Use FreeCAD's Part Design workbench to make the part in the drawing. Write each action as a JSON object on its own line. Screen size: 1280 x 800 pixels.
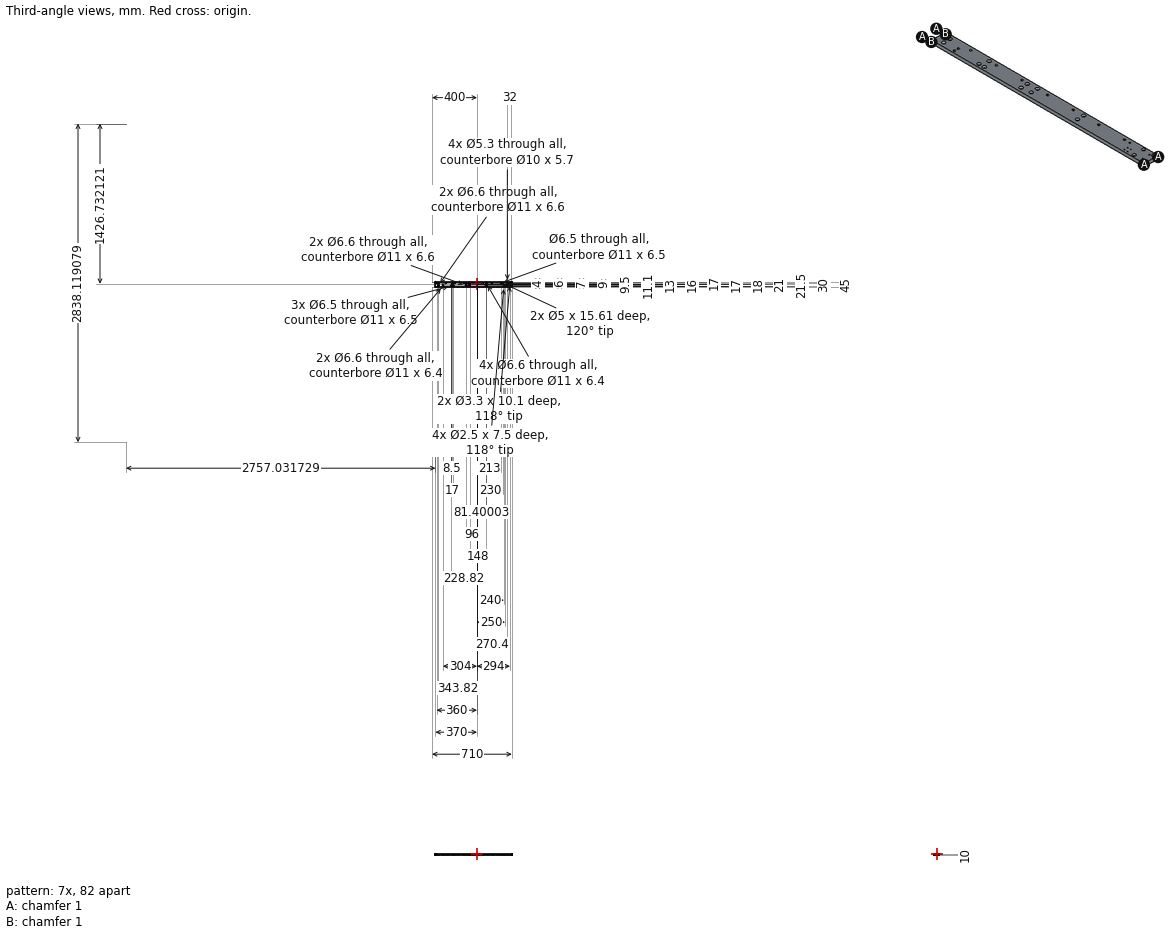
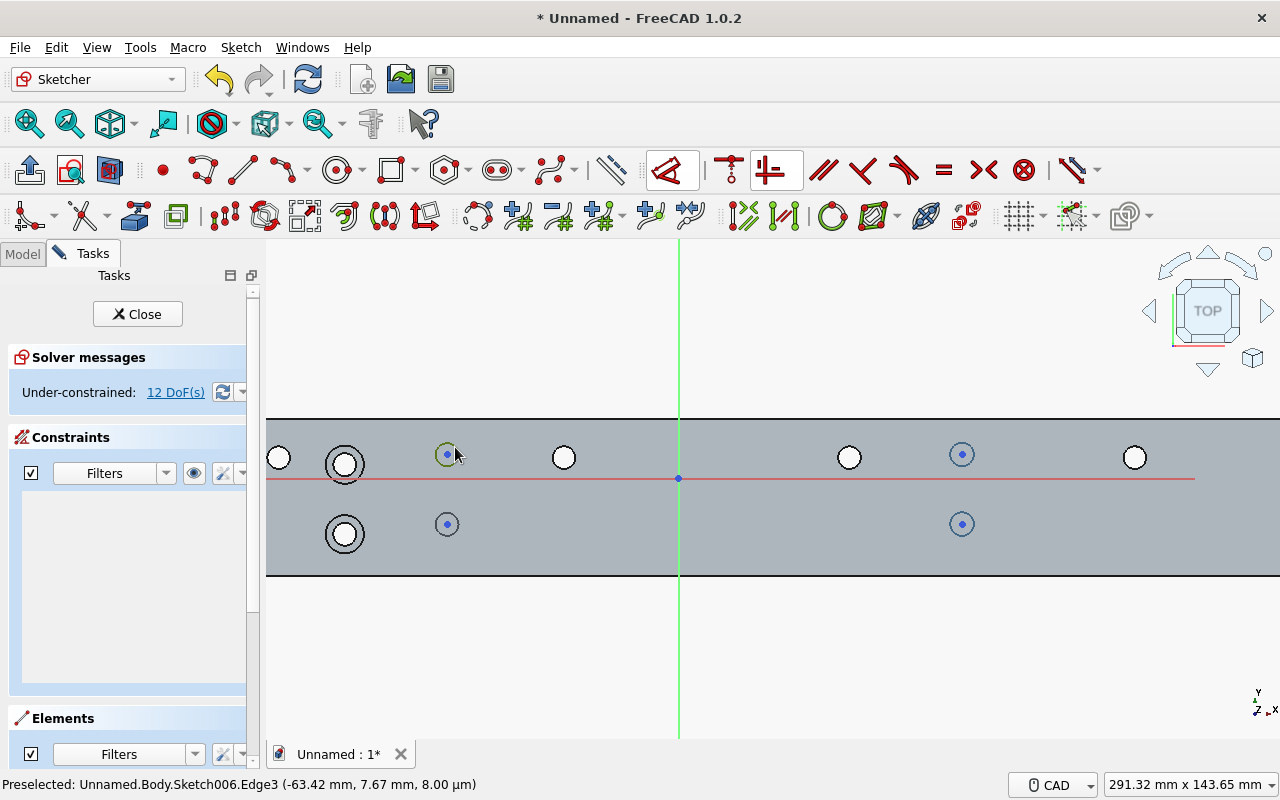
{"action": "left_click", "coordinate": [455, 516]}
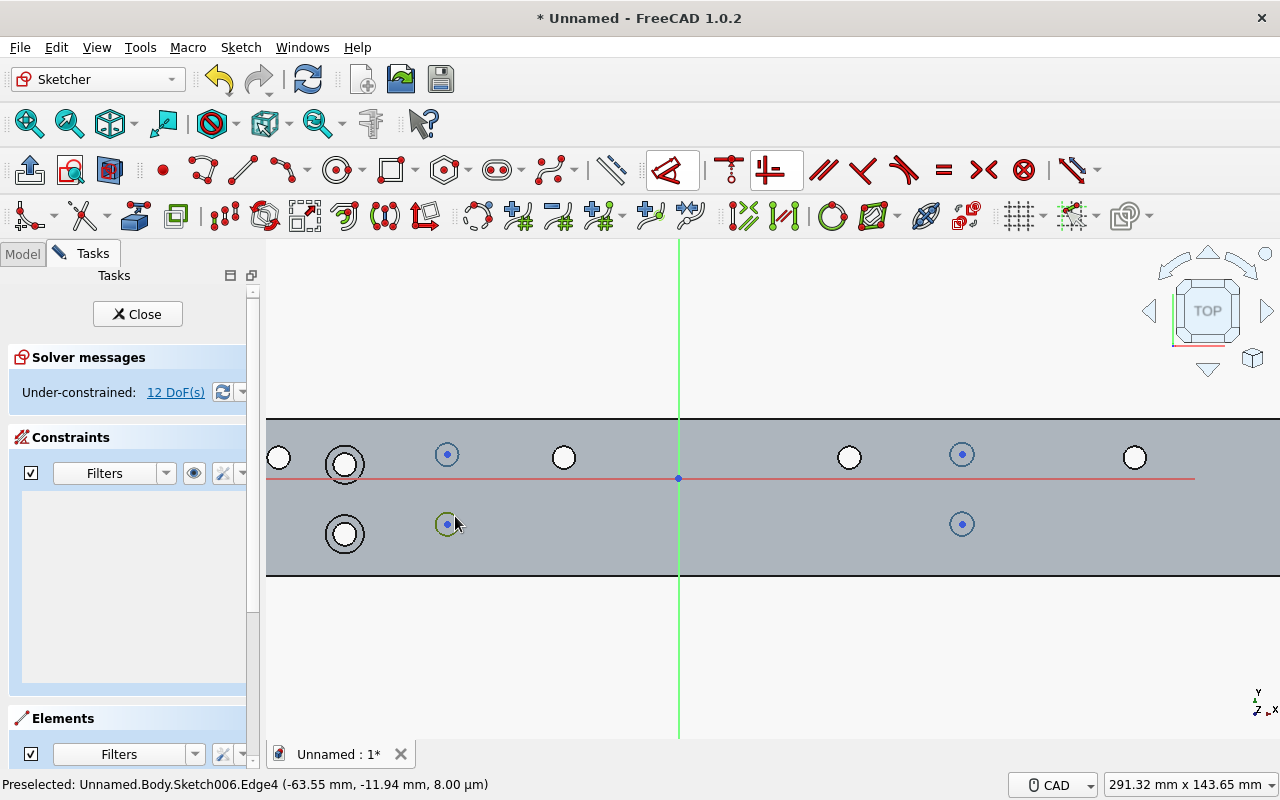
{"action": "left_click", "coordinate": [944, 170]}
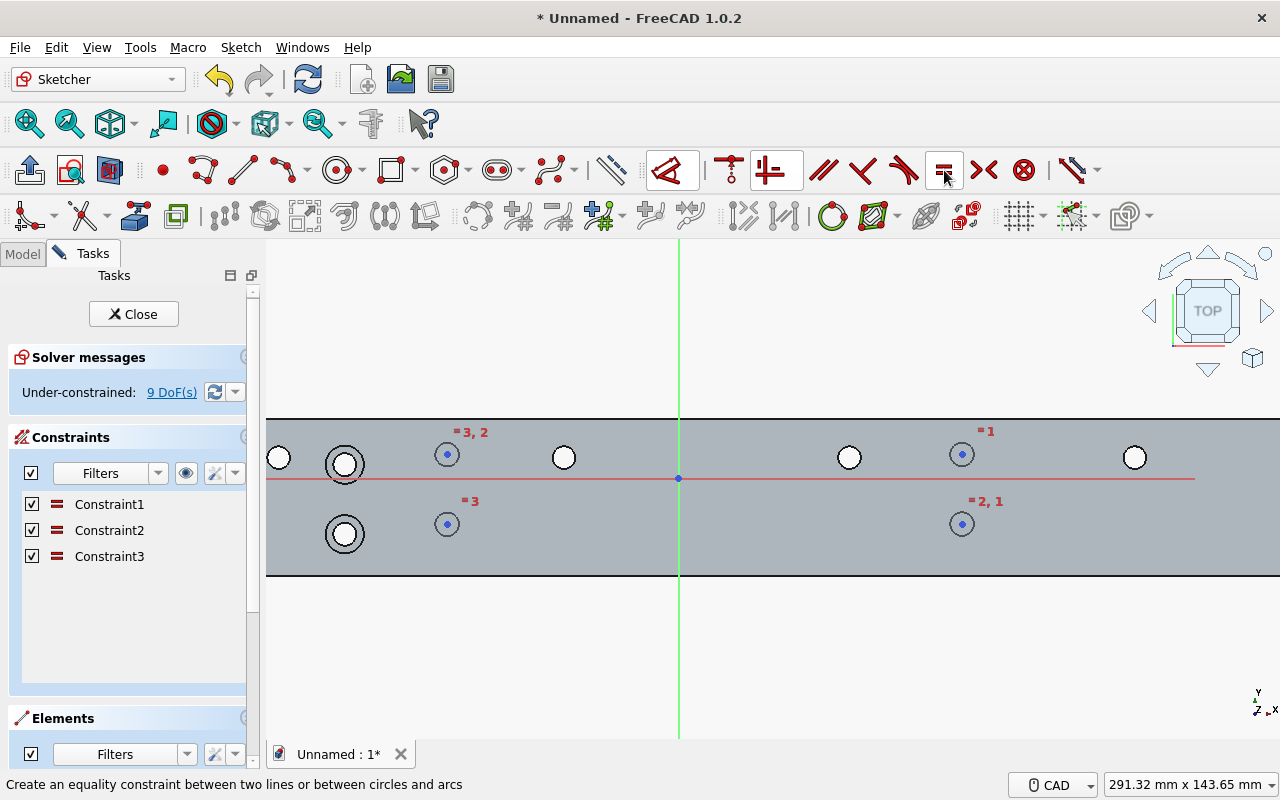
{"action": "left_click", "coordinate": [962, 454]}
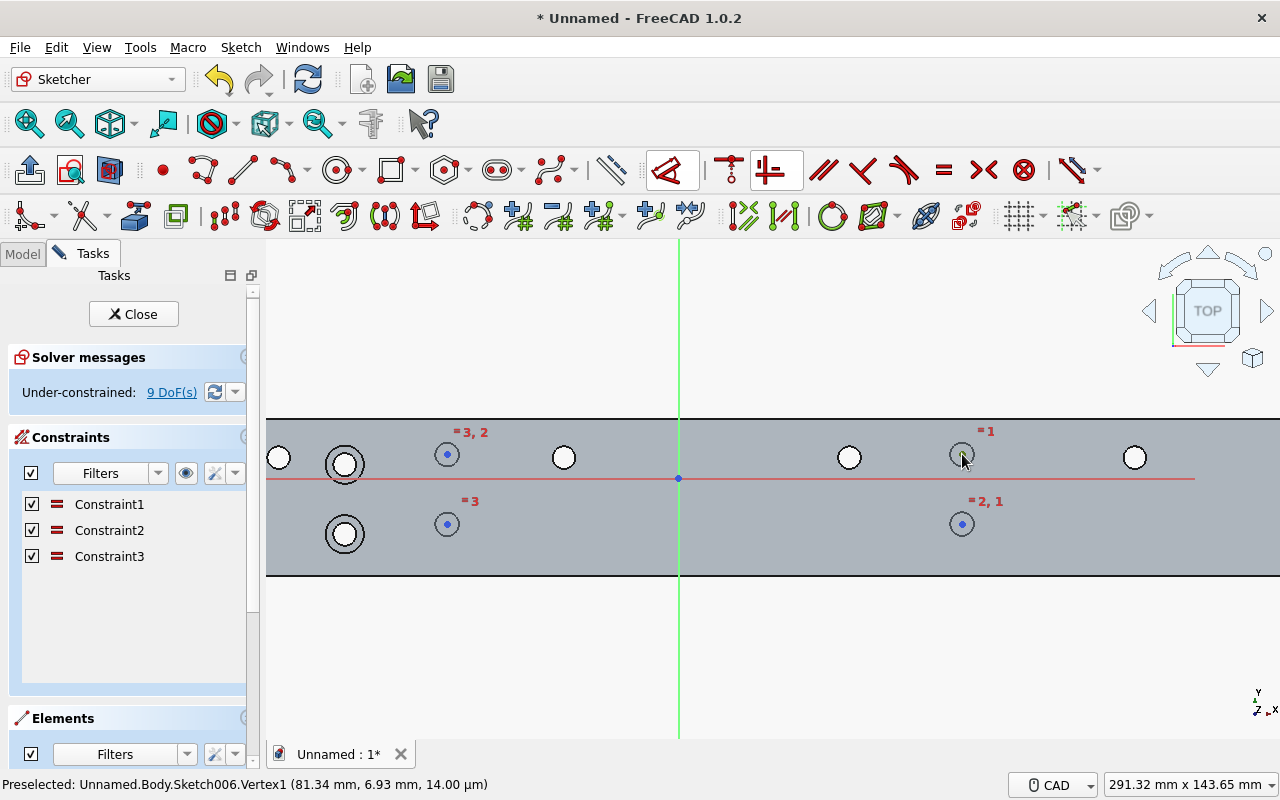
{"action": "left_click", "coordinate": [962, 524]}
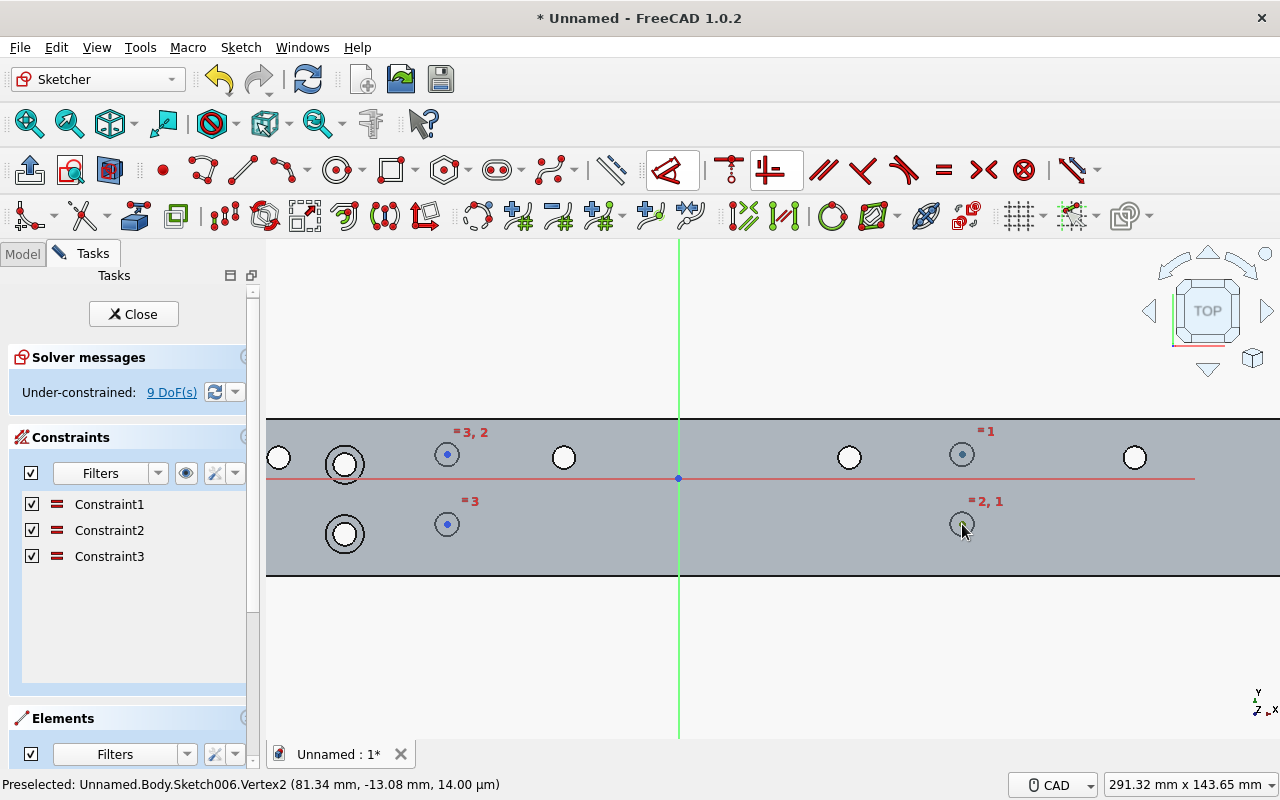
{"action": "left_click", "coordinate": [798, 170]}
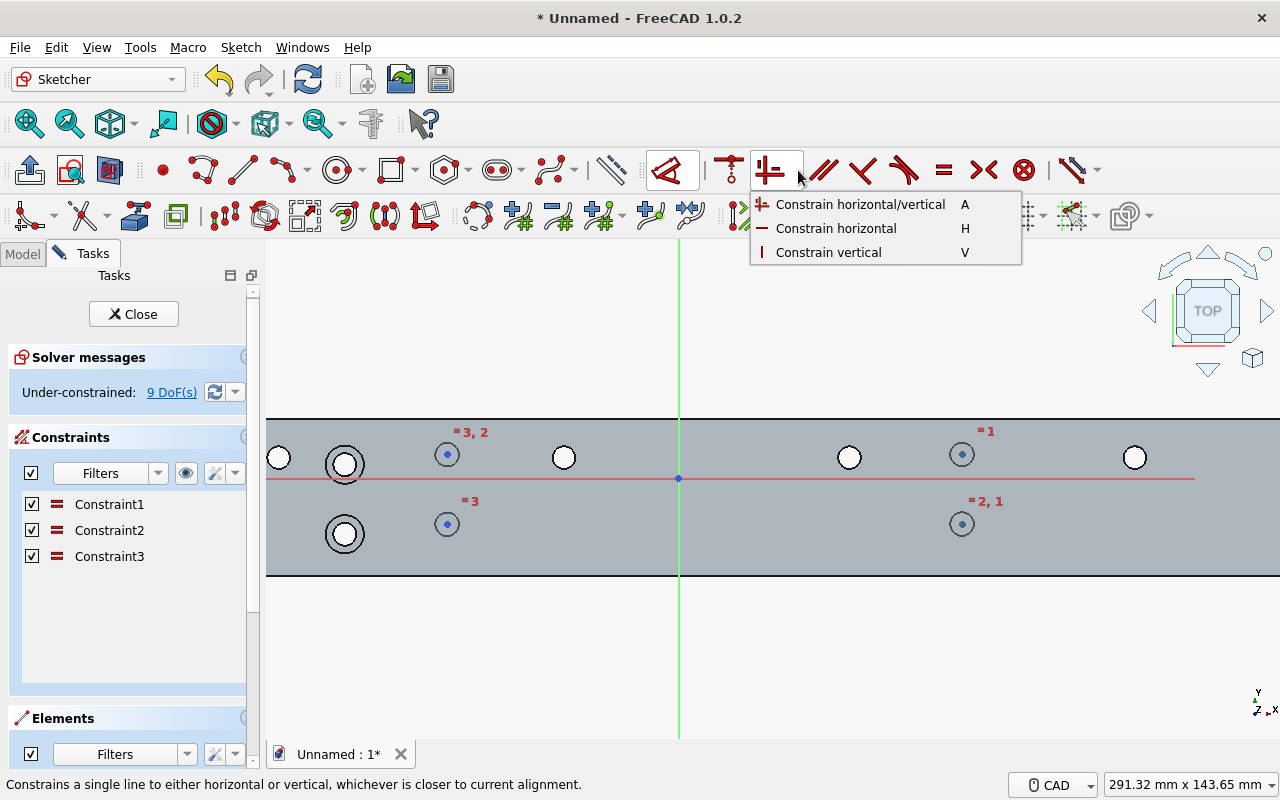
{"action": "left_click", "coordinate": [886, 252]}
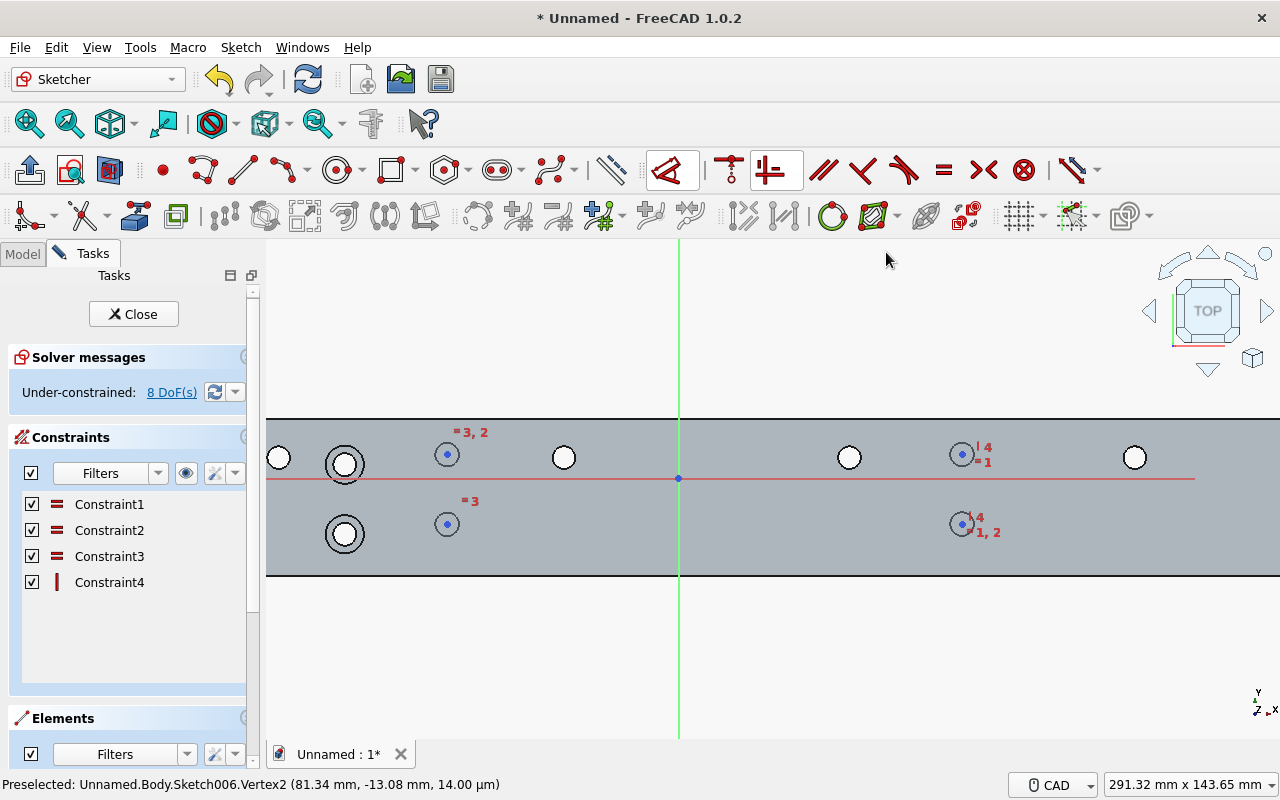
{"action": "left_click", "coordinate": [962, 454]}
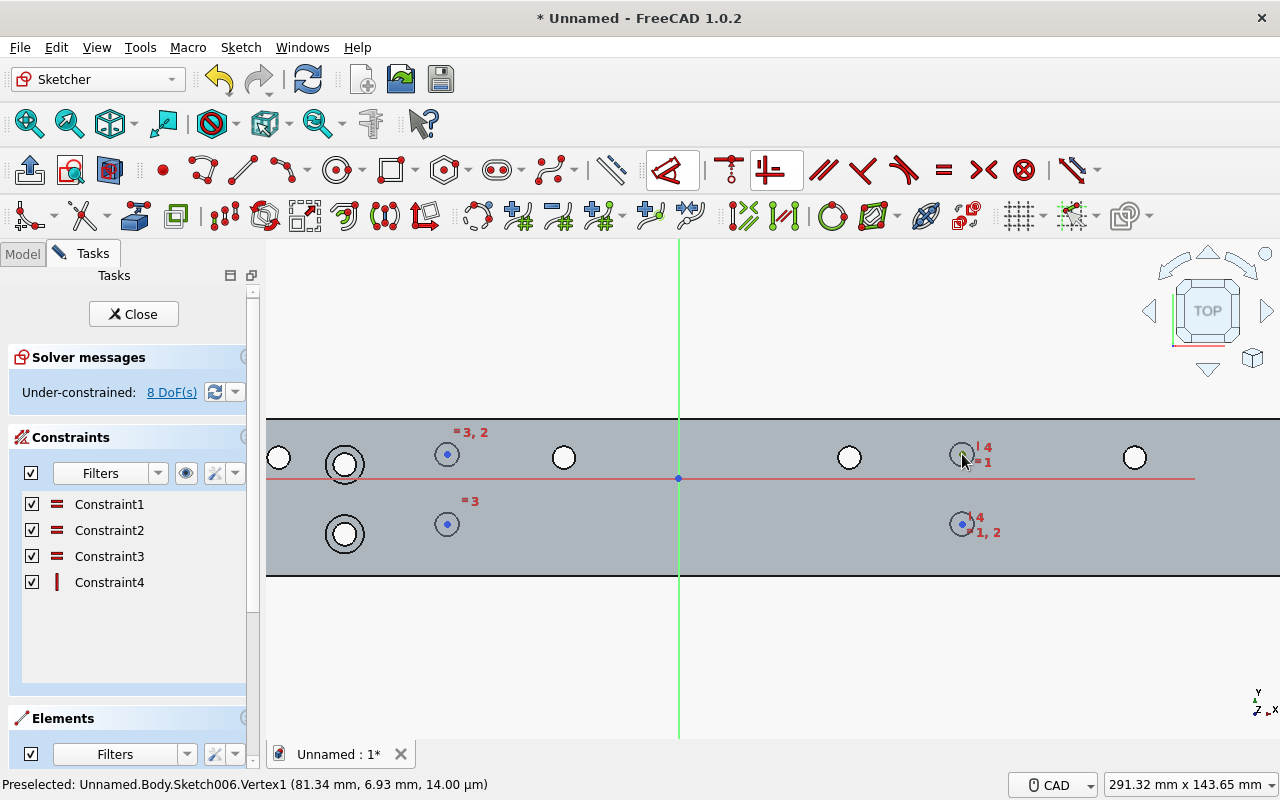
{"action": "left_click", "coordinate": [447, 455]}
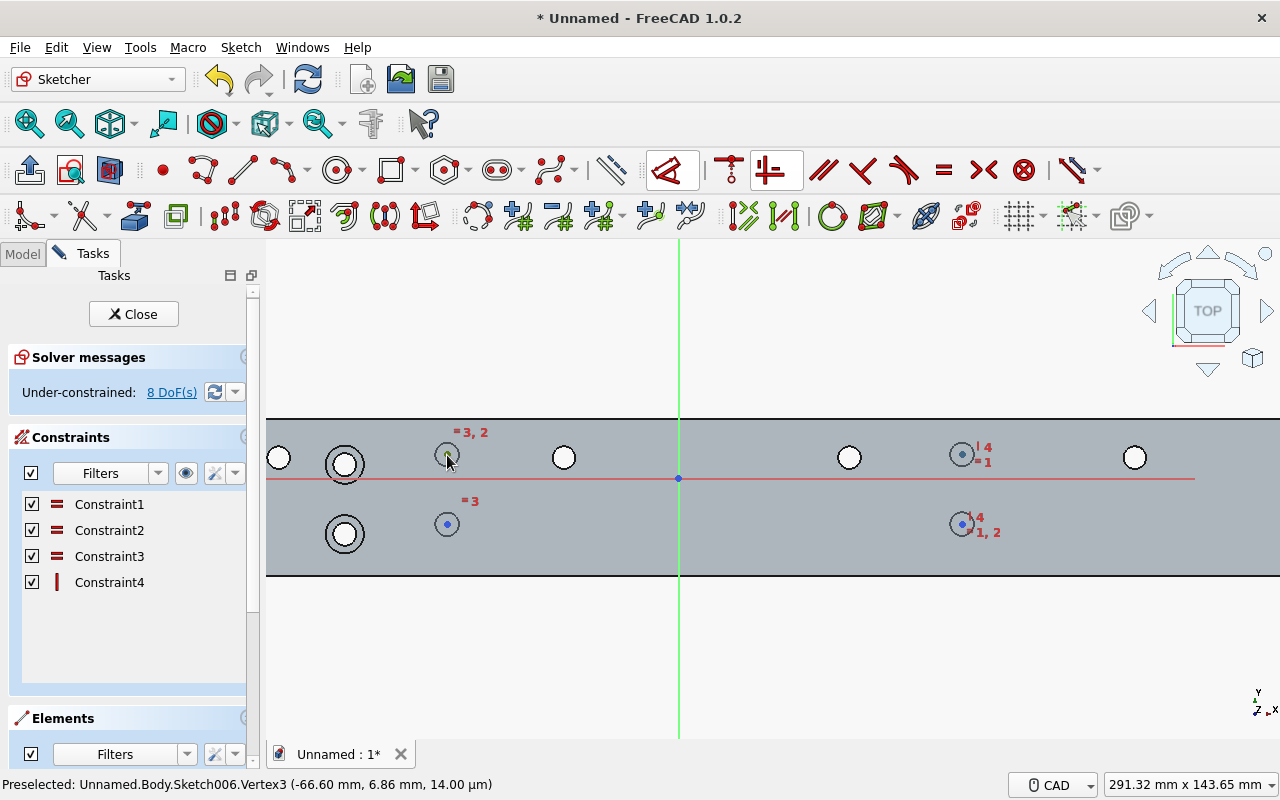
{"action": "left_click", "coordinate": [798, 170]}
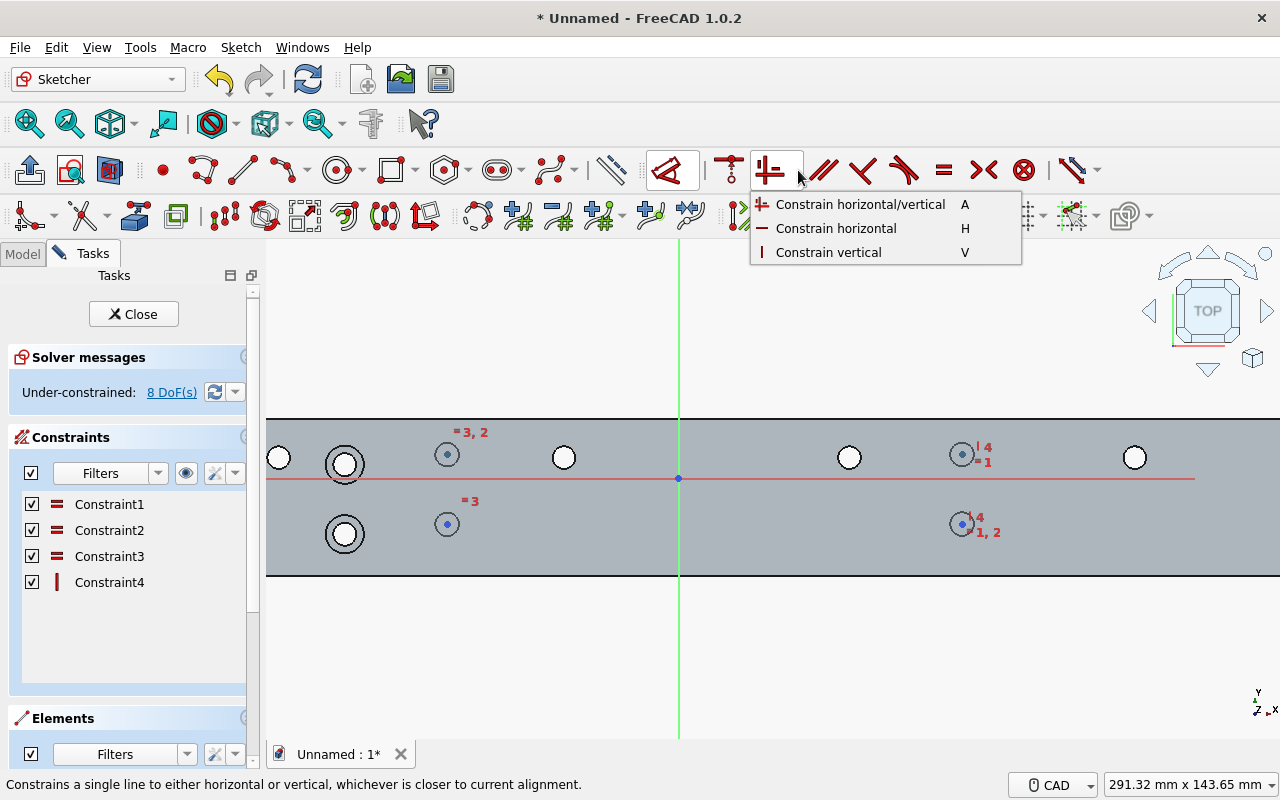
{"action": "left_click", "coordinate": [886, 228]}